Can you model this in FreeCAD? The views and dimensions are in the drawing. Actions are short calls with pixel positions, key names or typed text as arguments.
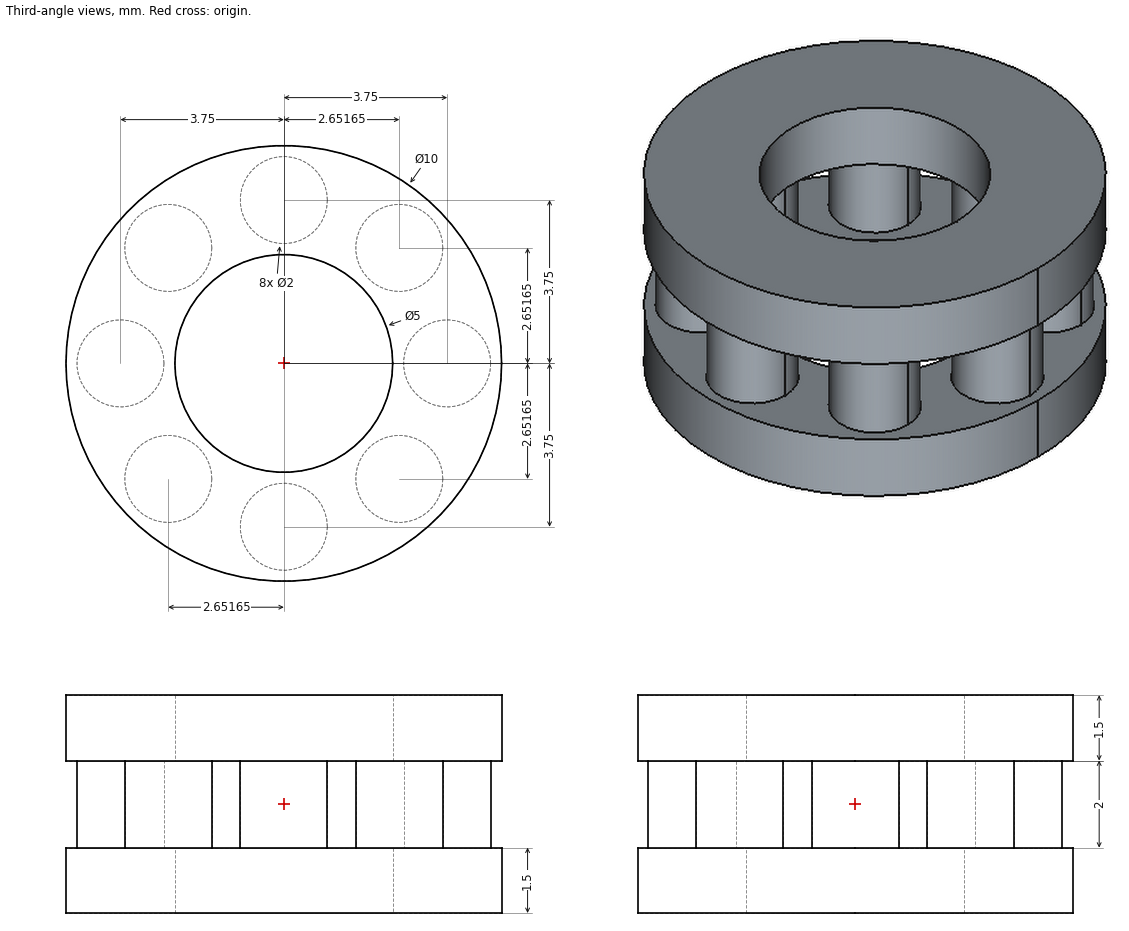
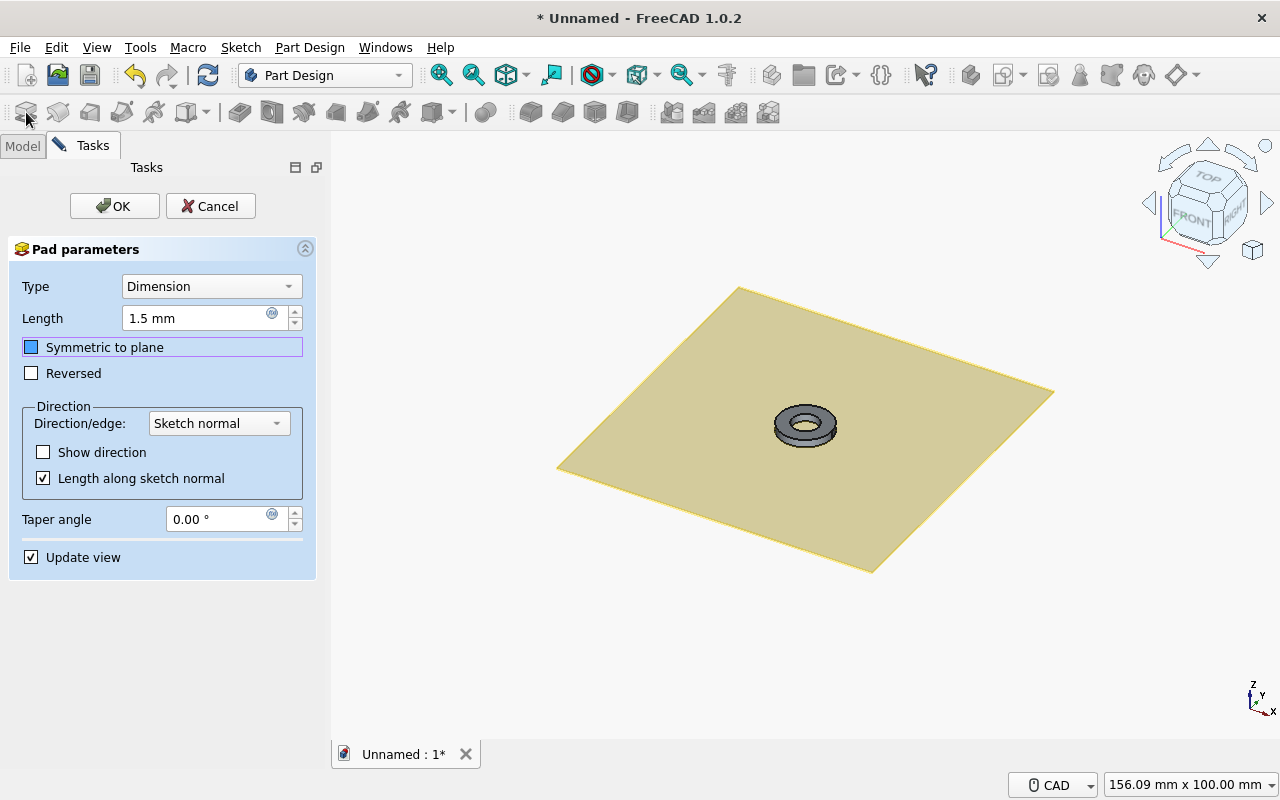
click(115, 206)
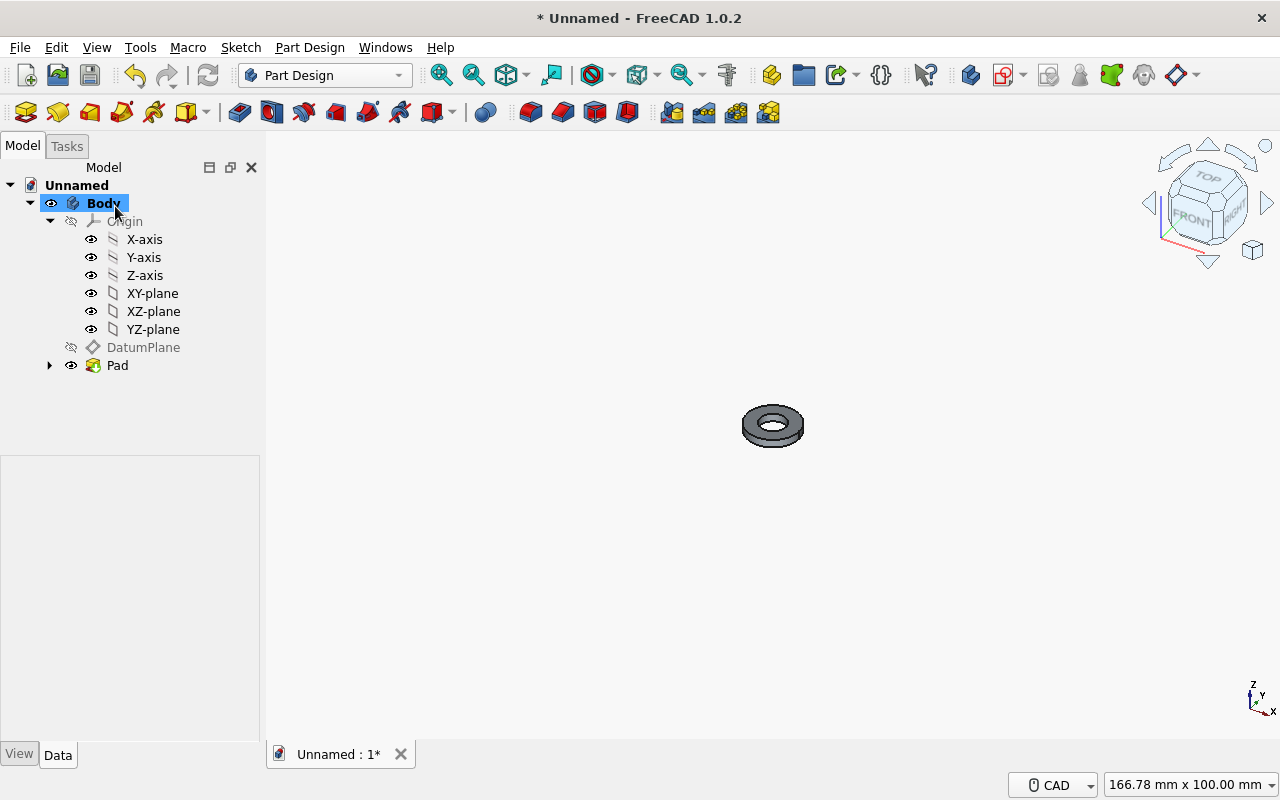
click(442, 76)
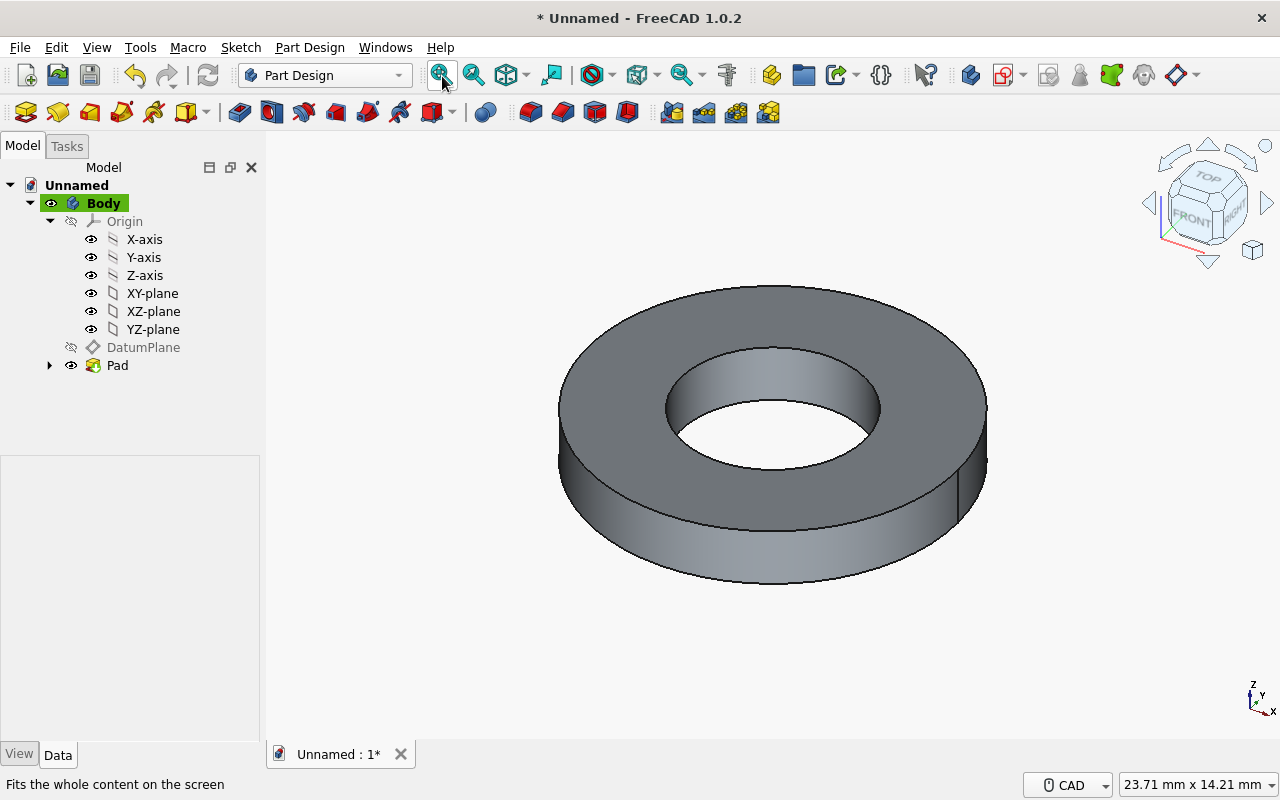
click(972, 76)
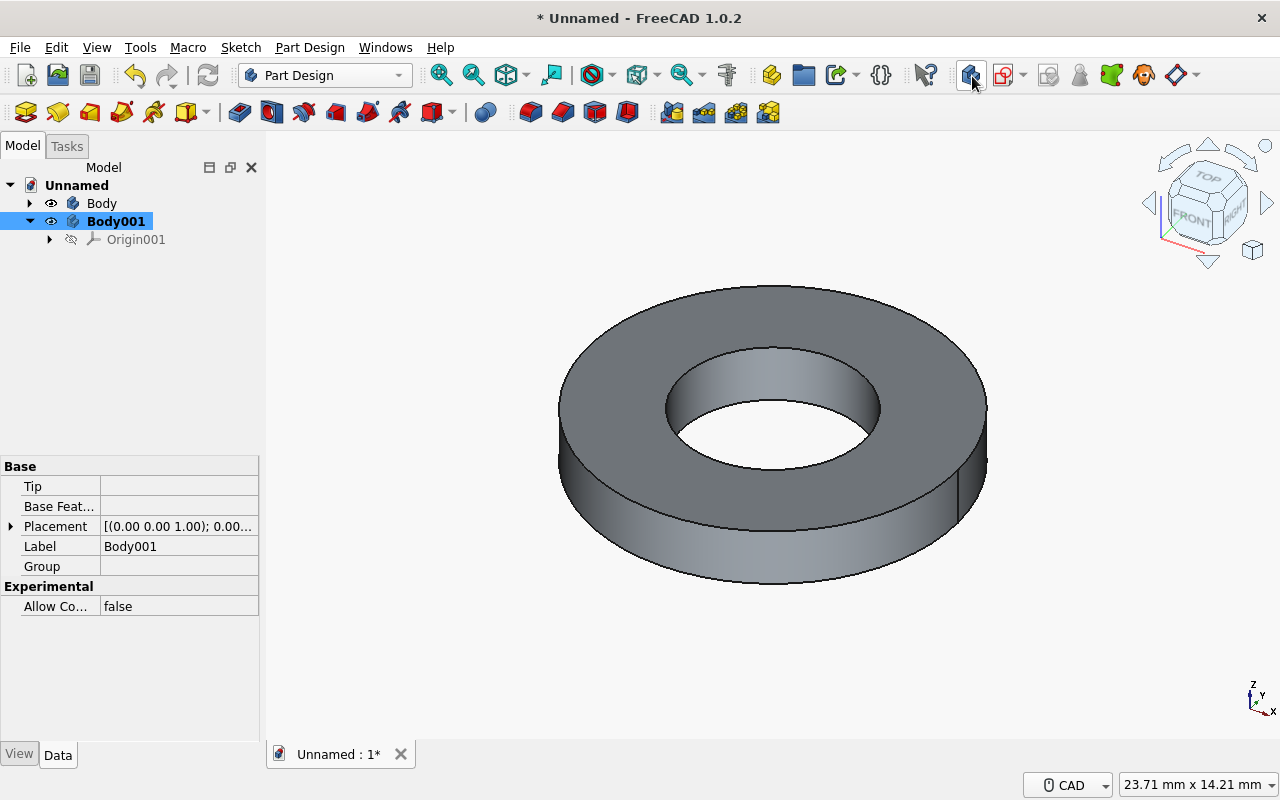
click(50, 239)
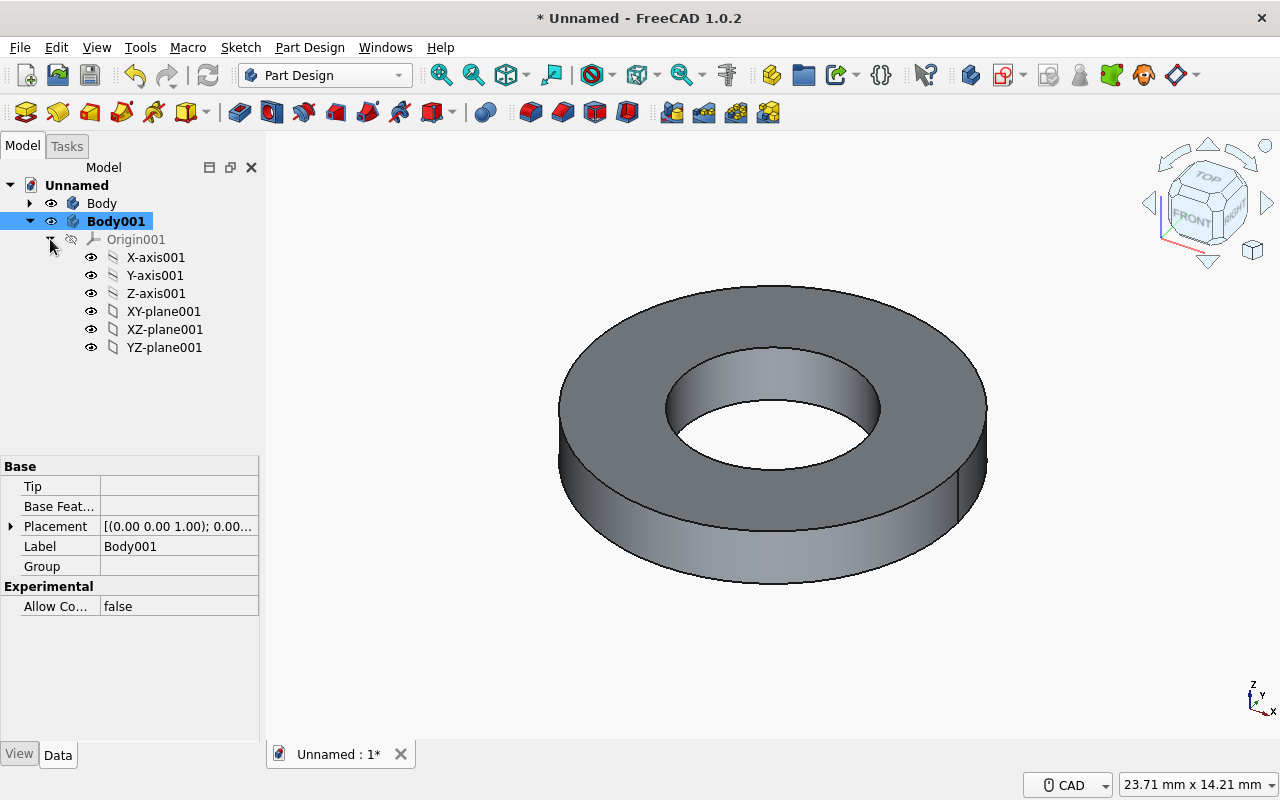
click(136, 311)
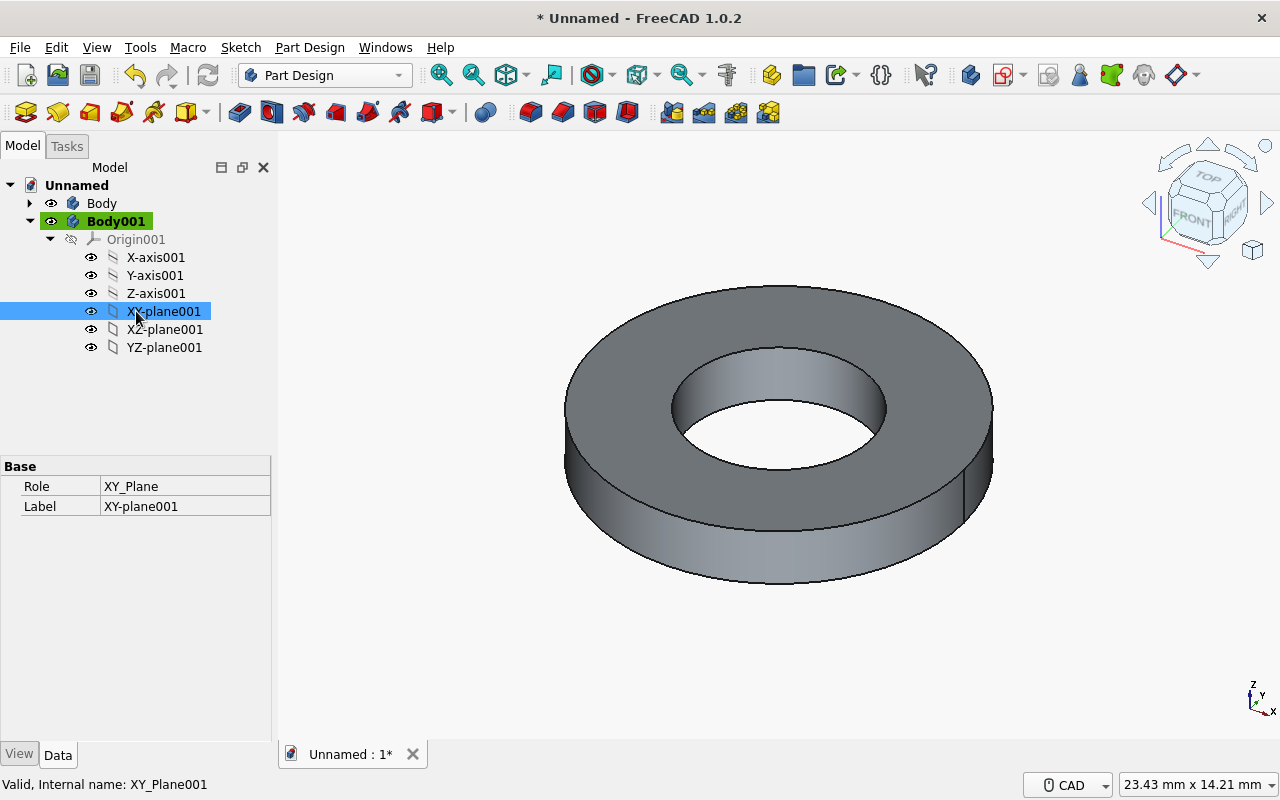
click(1176, 76)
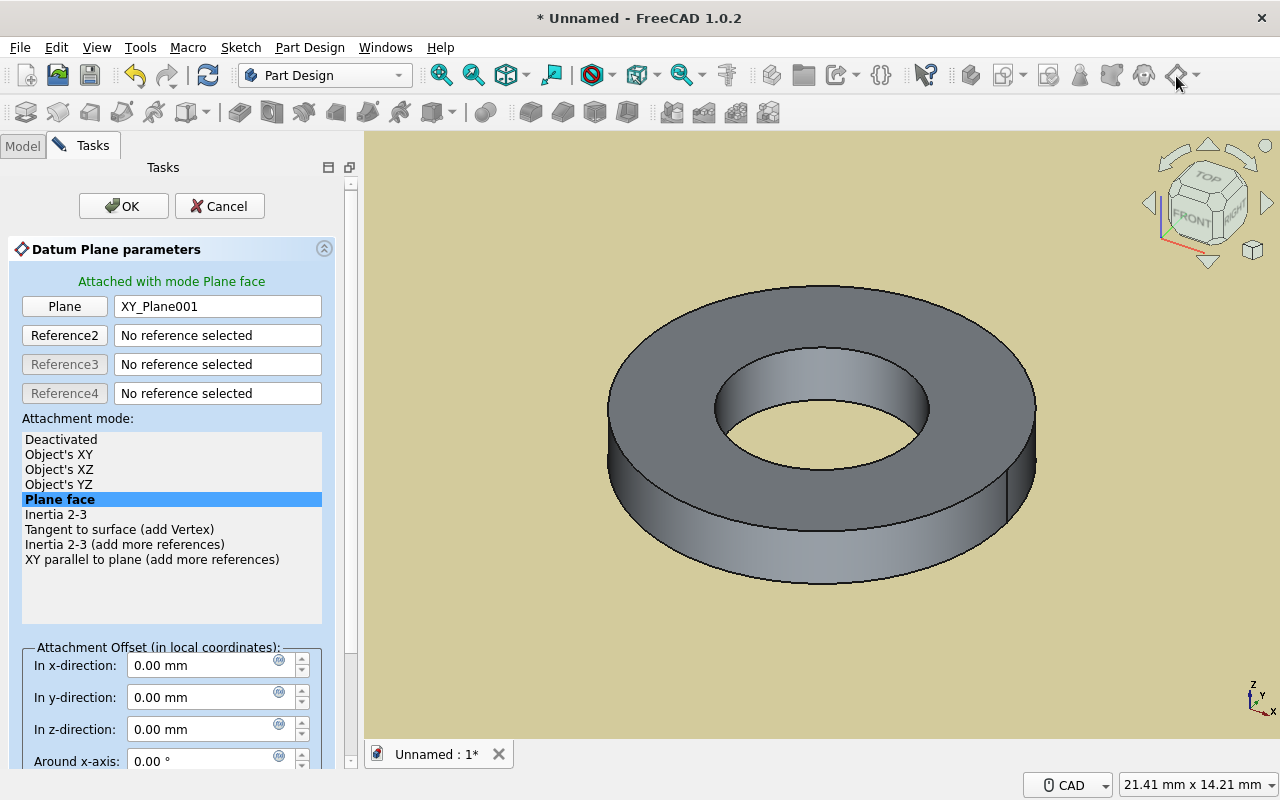
triple_click(210, 729)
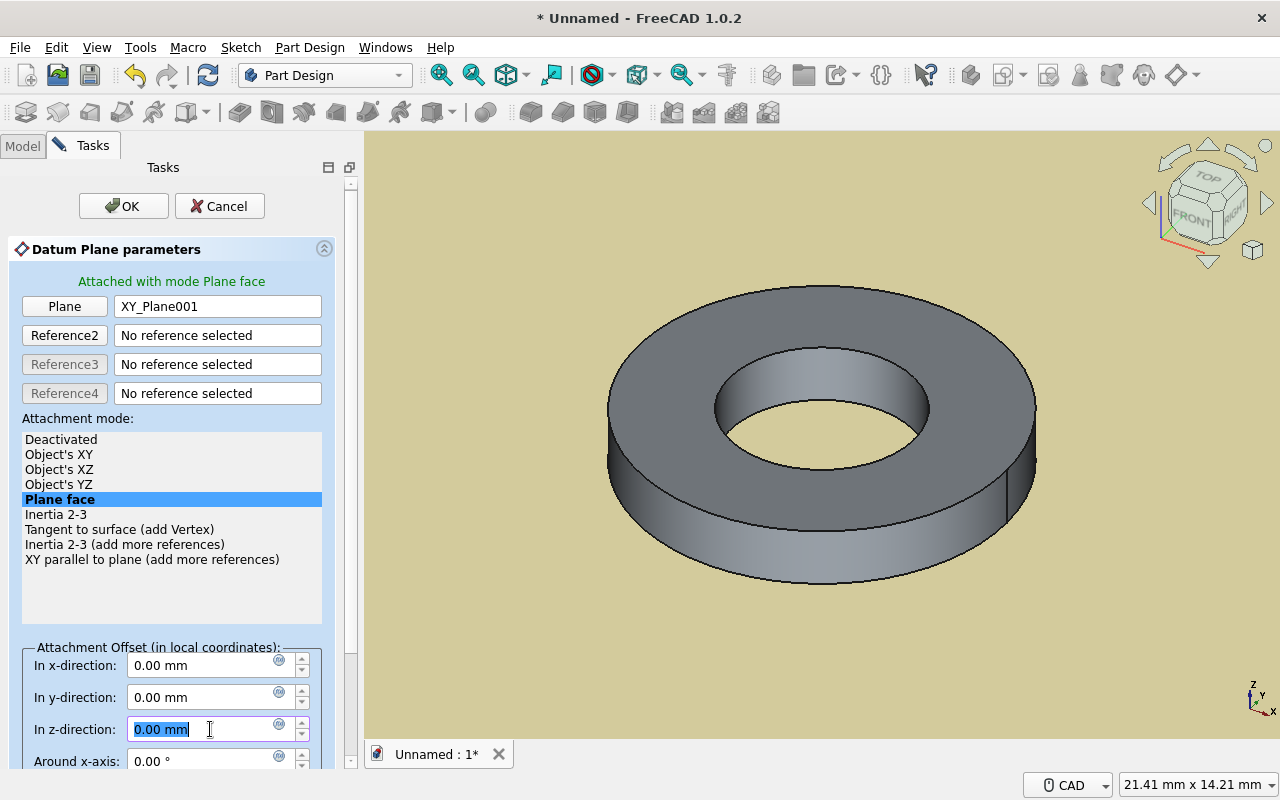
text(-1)
key(Tab)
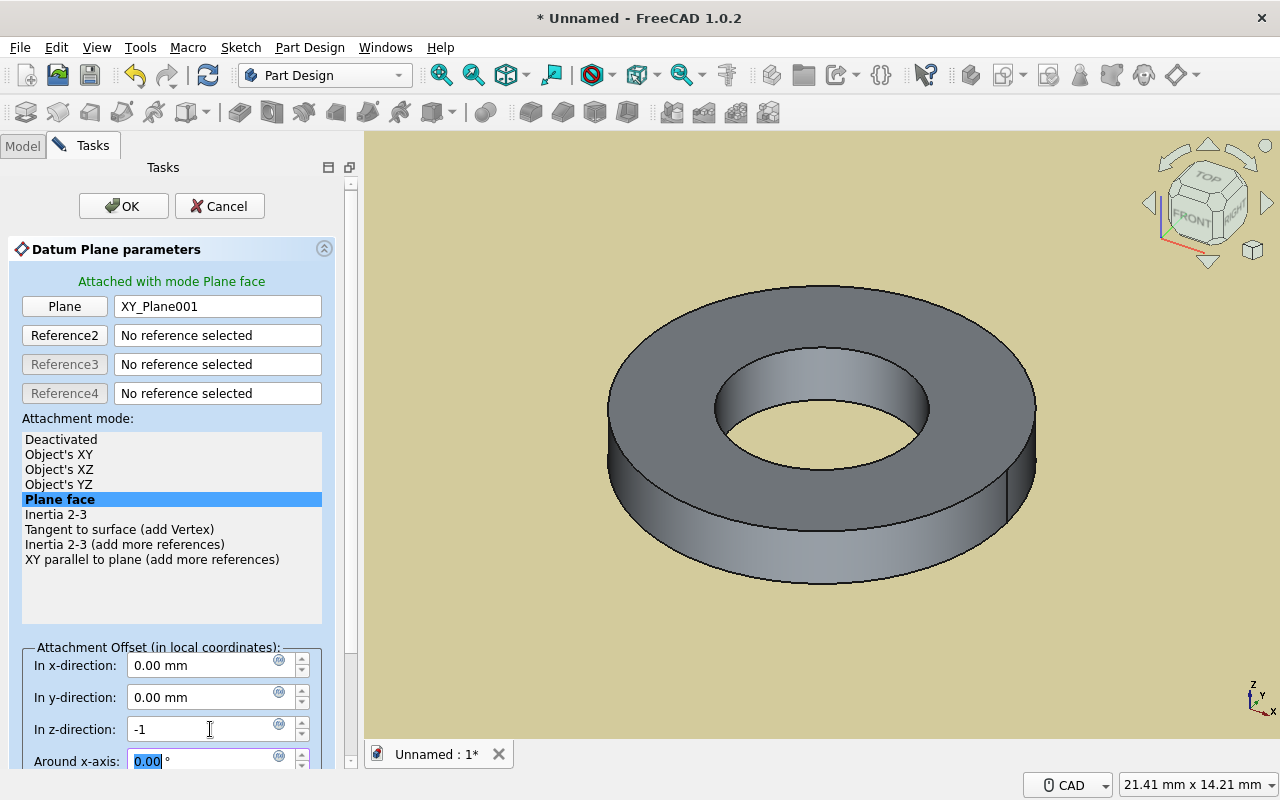
click(124, 206)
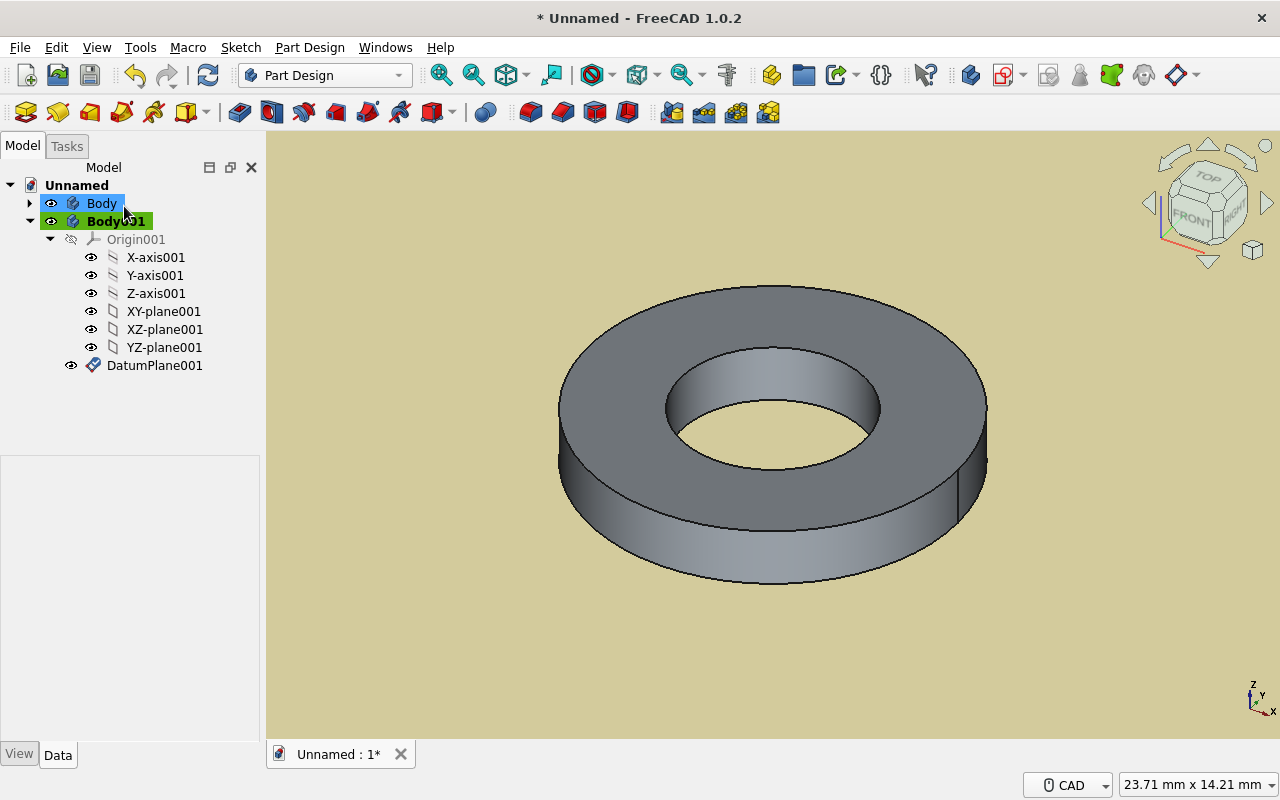
click(116, 365)